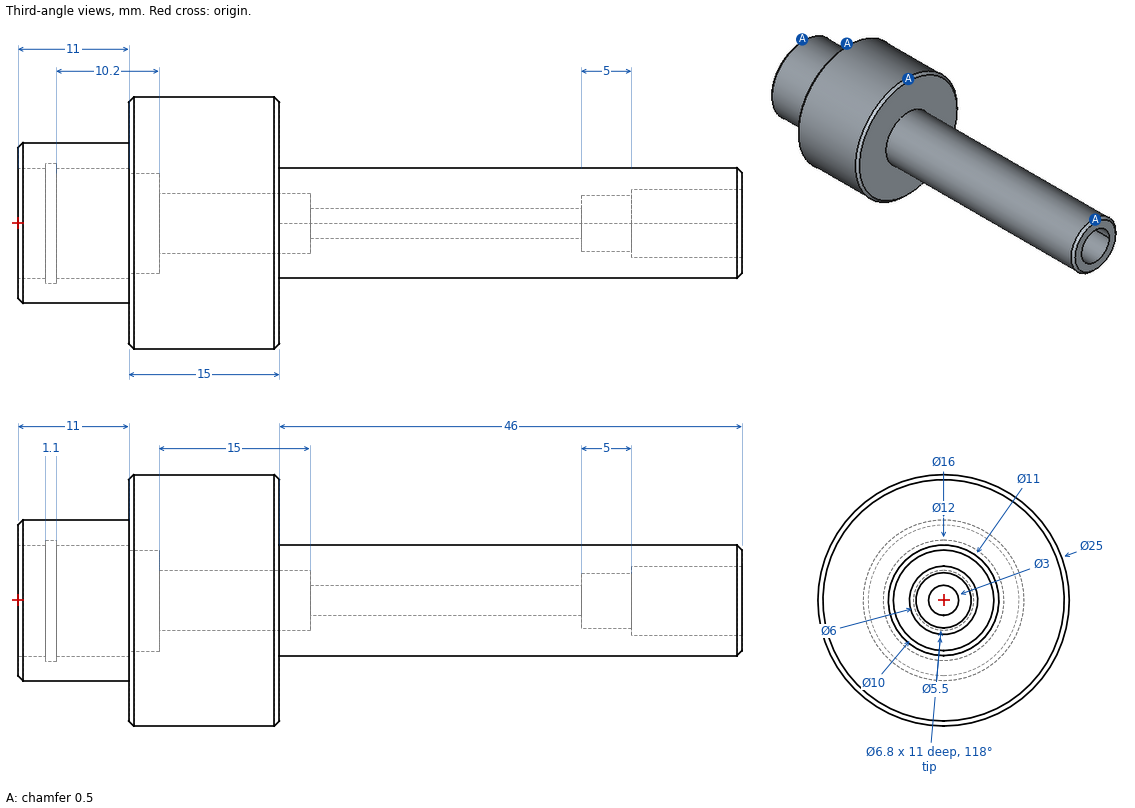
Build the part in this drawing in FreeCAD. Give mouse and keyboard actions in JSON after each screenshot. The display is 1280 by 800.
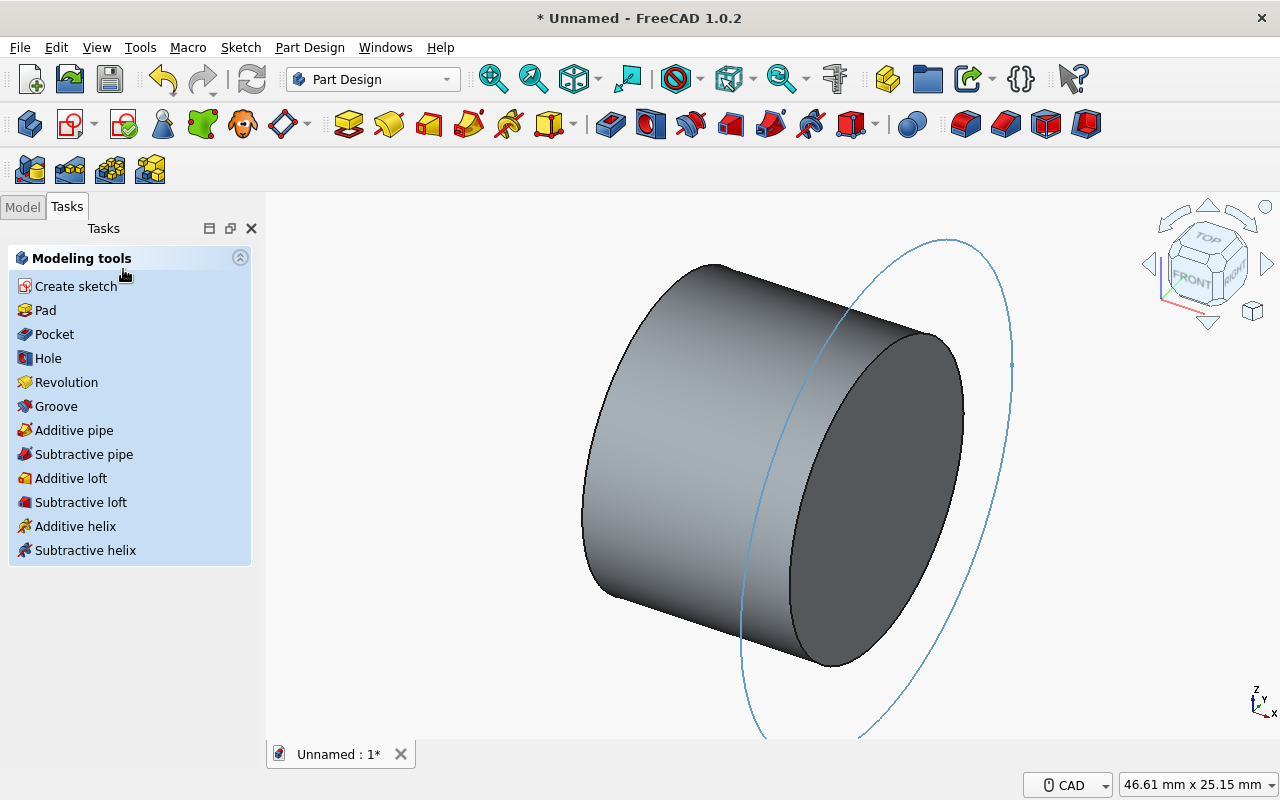
{"action": "left_click", "coordinate": [350, 124]}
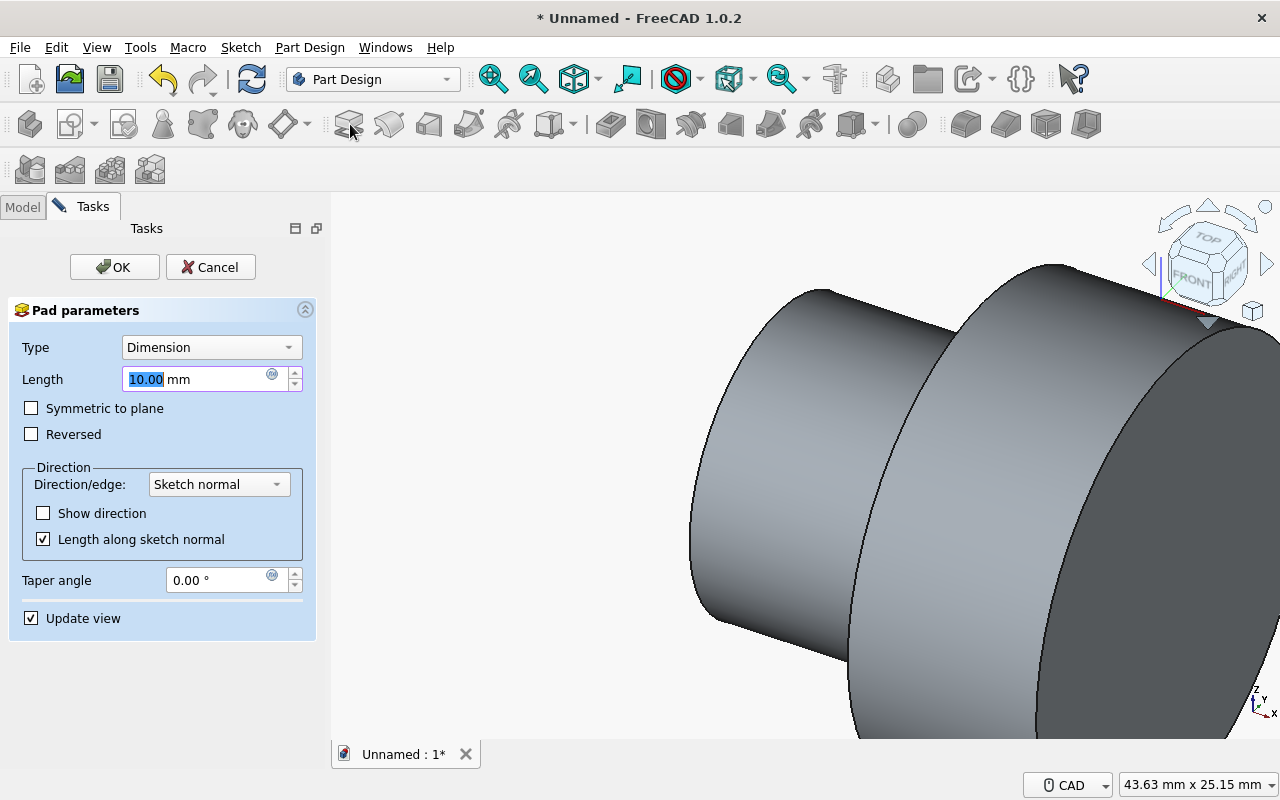
{"action": "type", "text": "15"}
{"action": "key", "text": "Tab"}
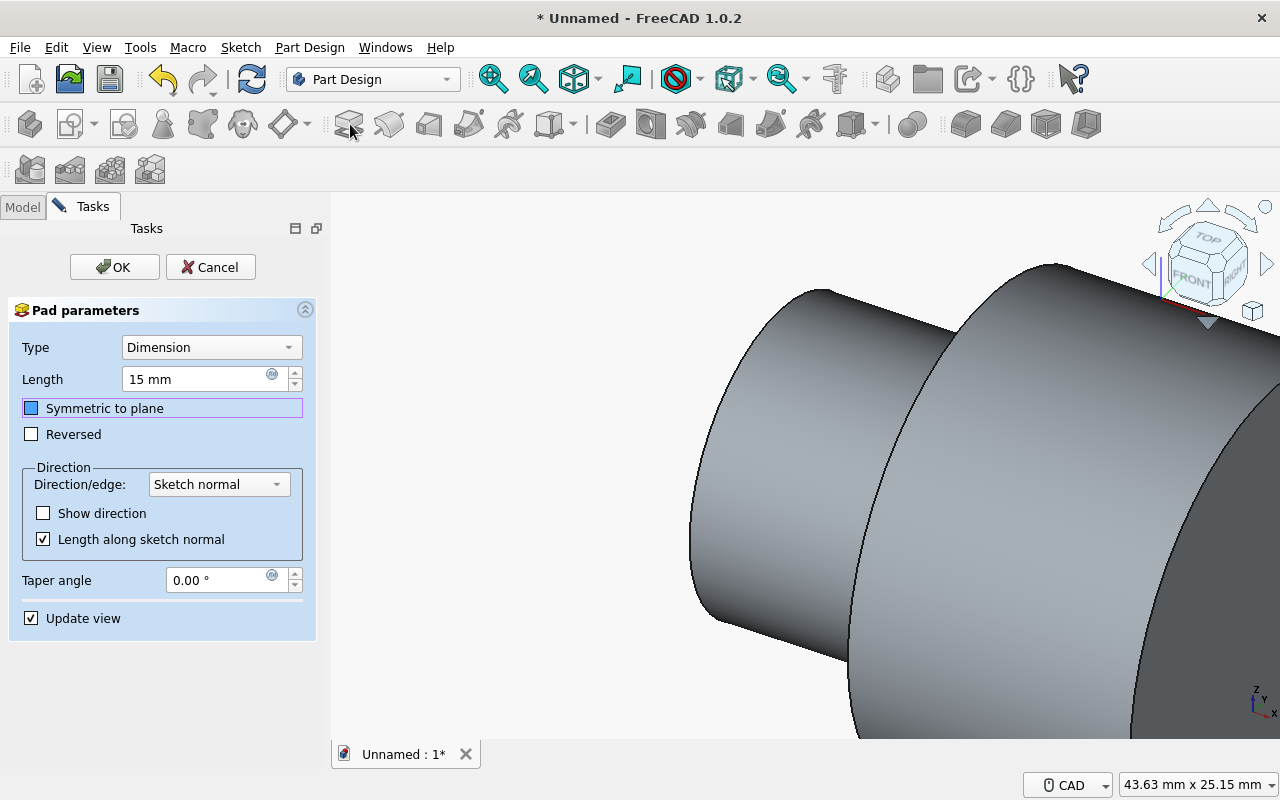
{"action": "left_click", "coordinate": [115, 267]}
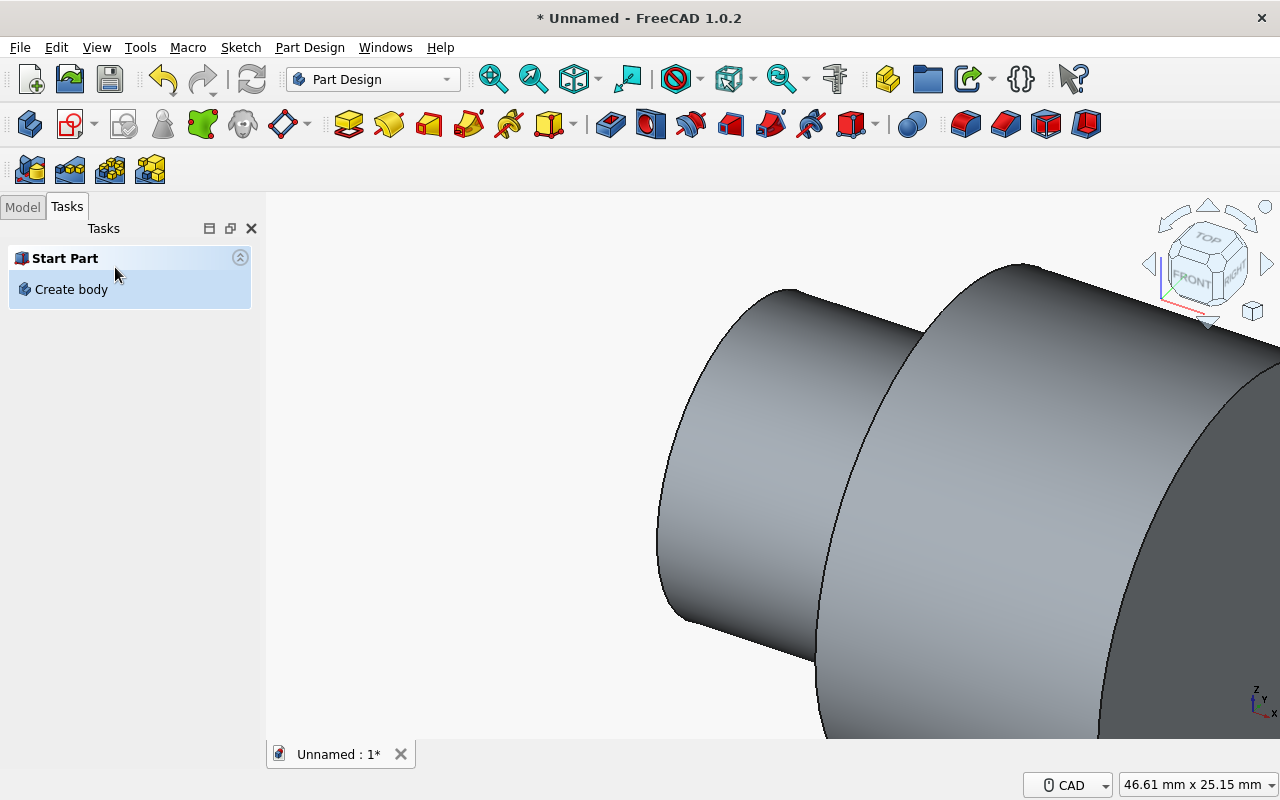
{"action": "left_click", "coordinate": [494, 80]}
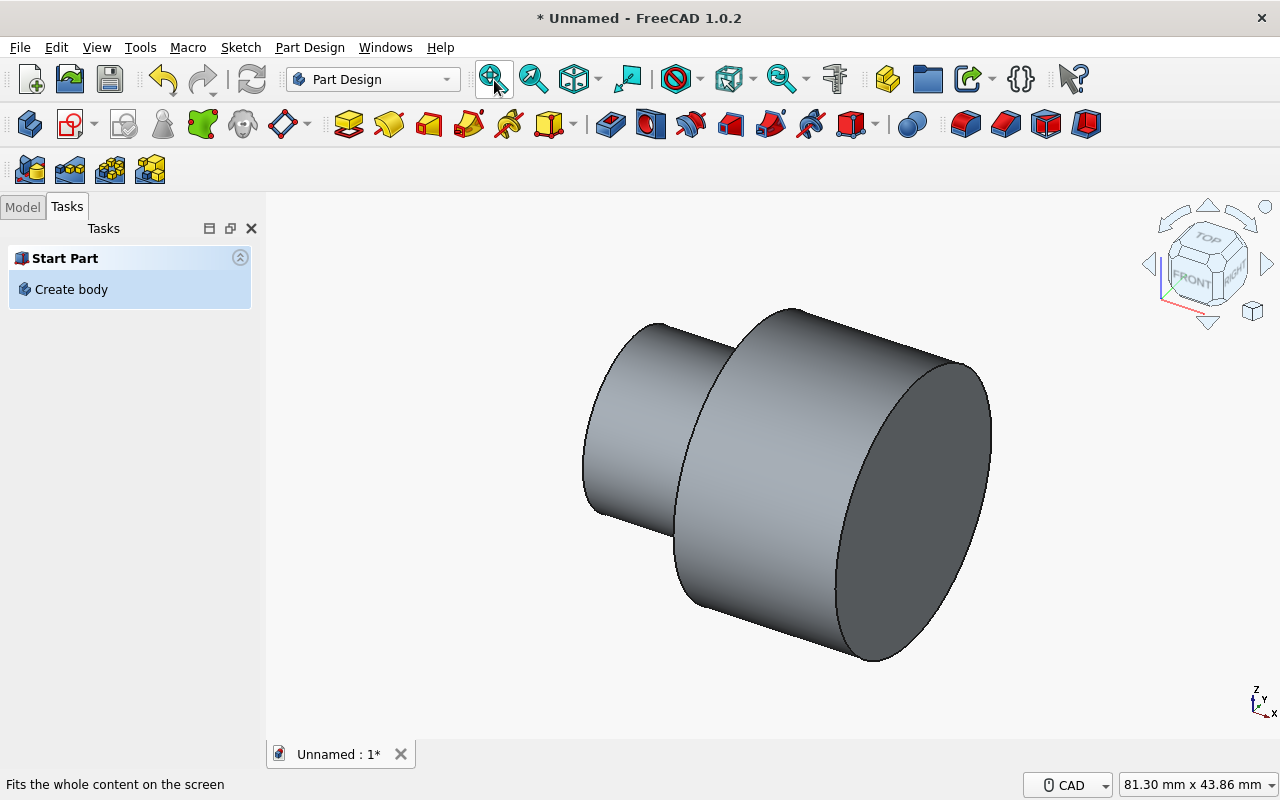
{"action": "left_click", "coordinate": [913, 511]}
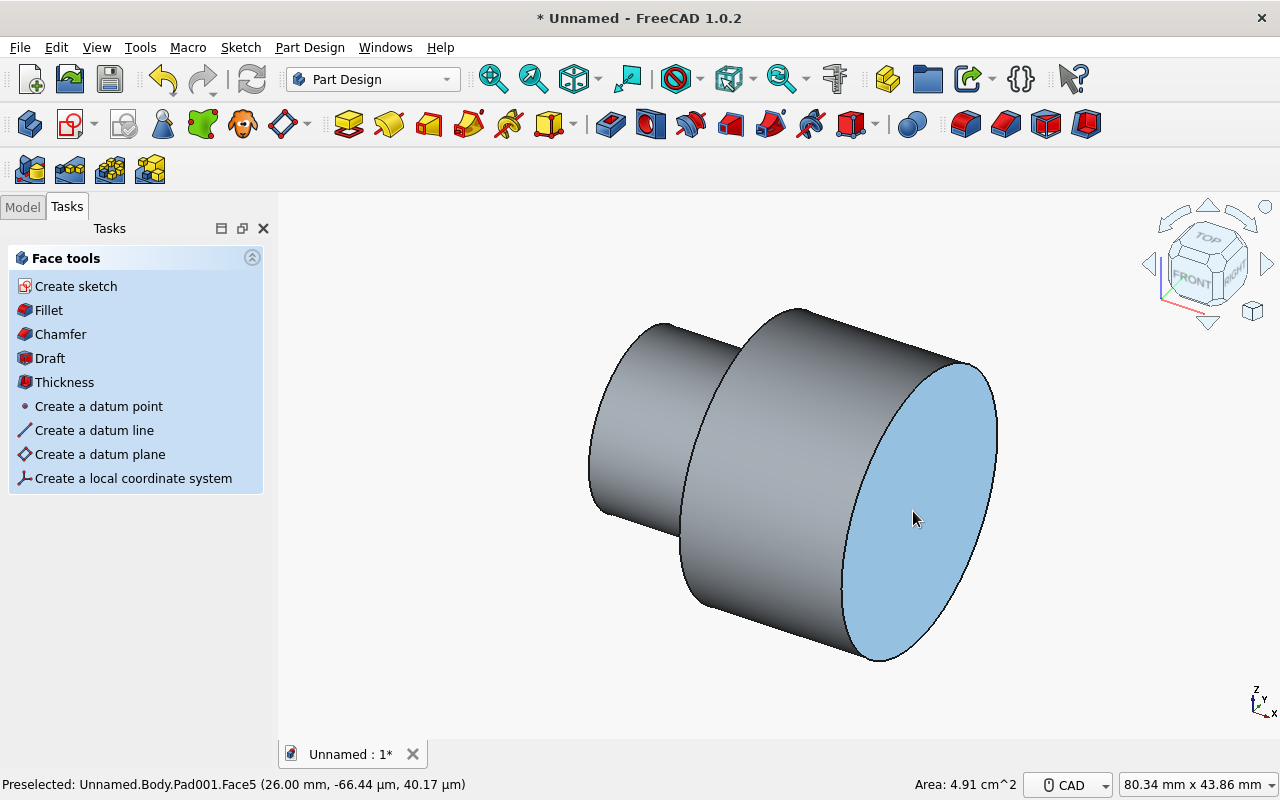
{"action": "left_click", "coordinate": [70, 124]}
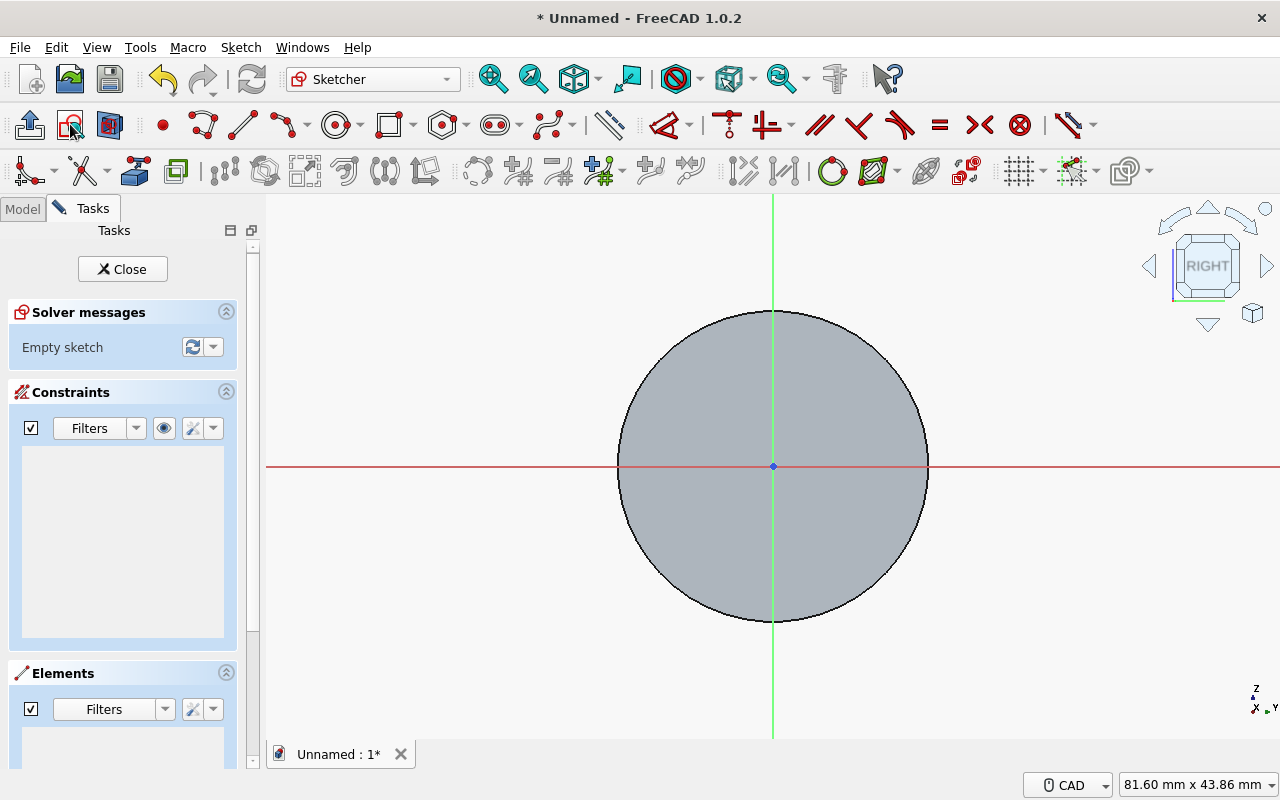
{"action": "scroll", "coordinate": [813, 466], "scroll_direction": "up", "scroll_amount": 5}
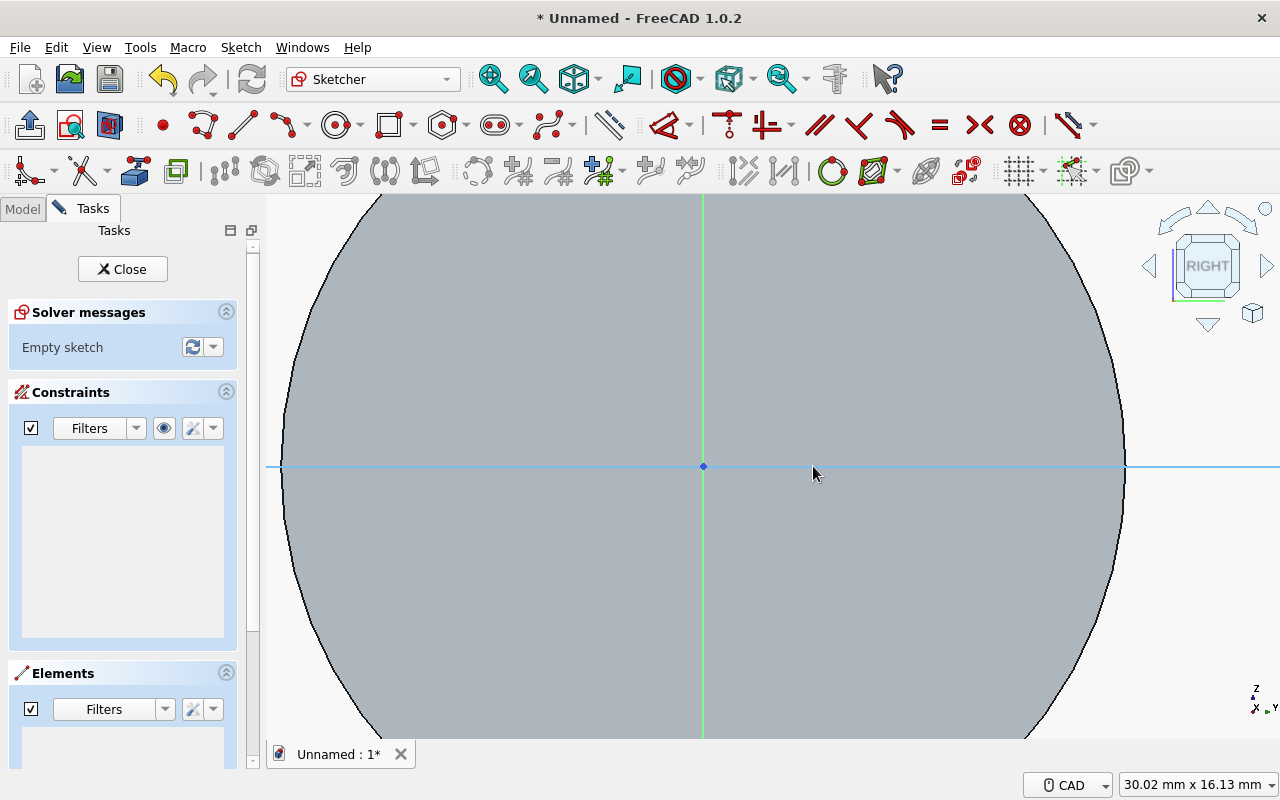
{"action": "left_click", "coordinate": [336, 126]}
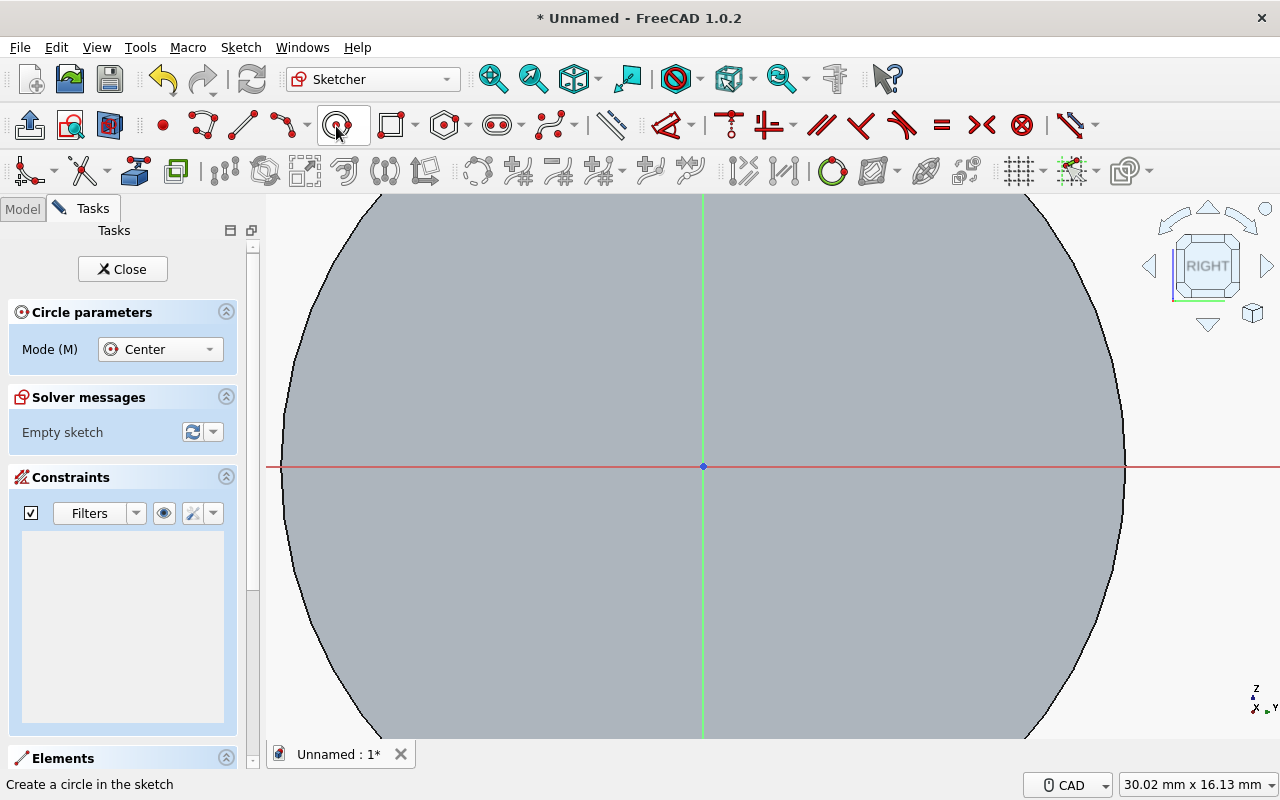
{"action": "left_click", "coordinate": [703, 466]}
{"action": "mouse_move", "coordinate": [835, 335]}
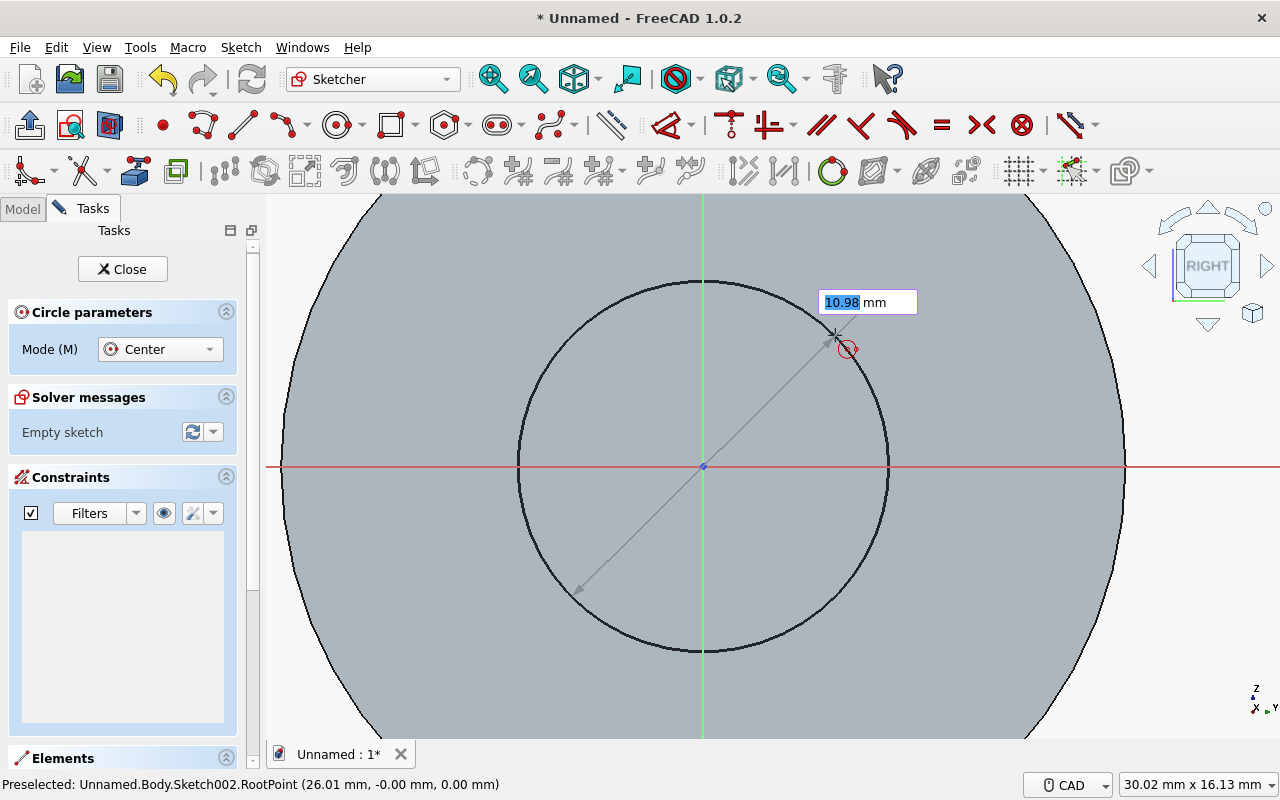
{"action": "type", "text": "11"}
{"action": "key", "text": "Return"}
{"action": "key", "text": "Escape"}